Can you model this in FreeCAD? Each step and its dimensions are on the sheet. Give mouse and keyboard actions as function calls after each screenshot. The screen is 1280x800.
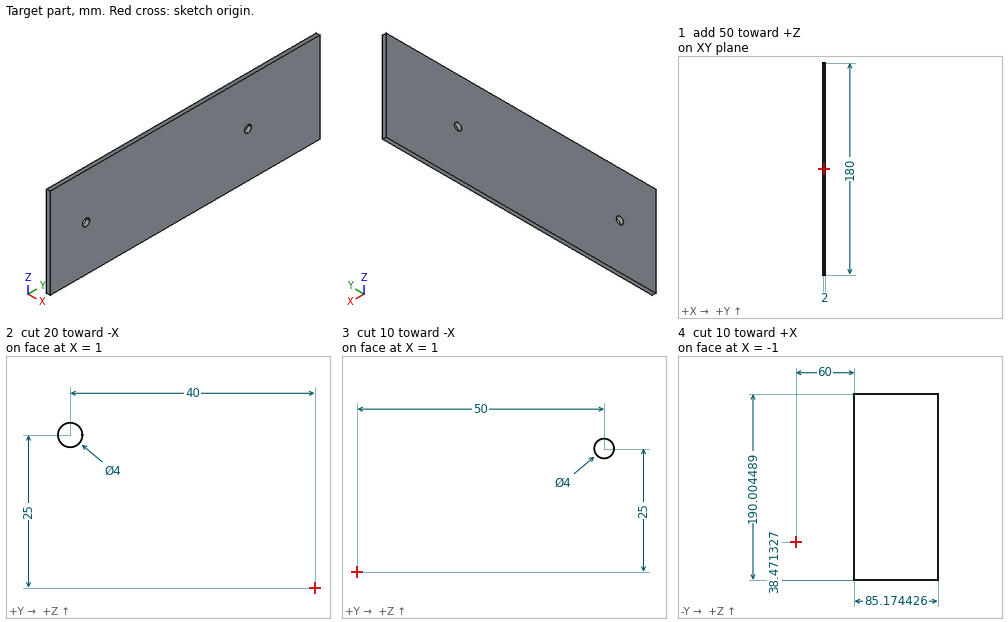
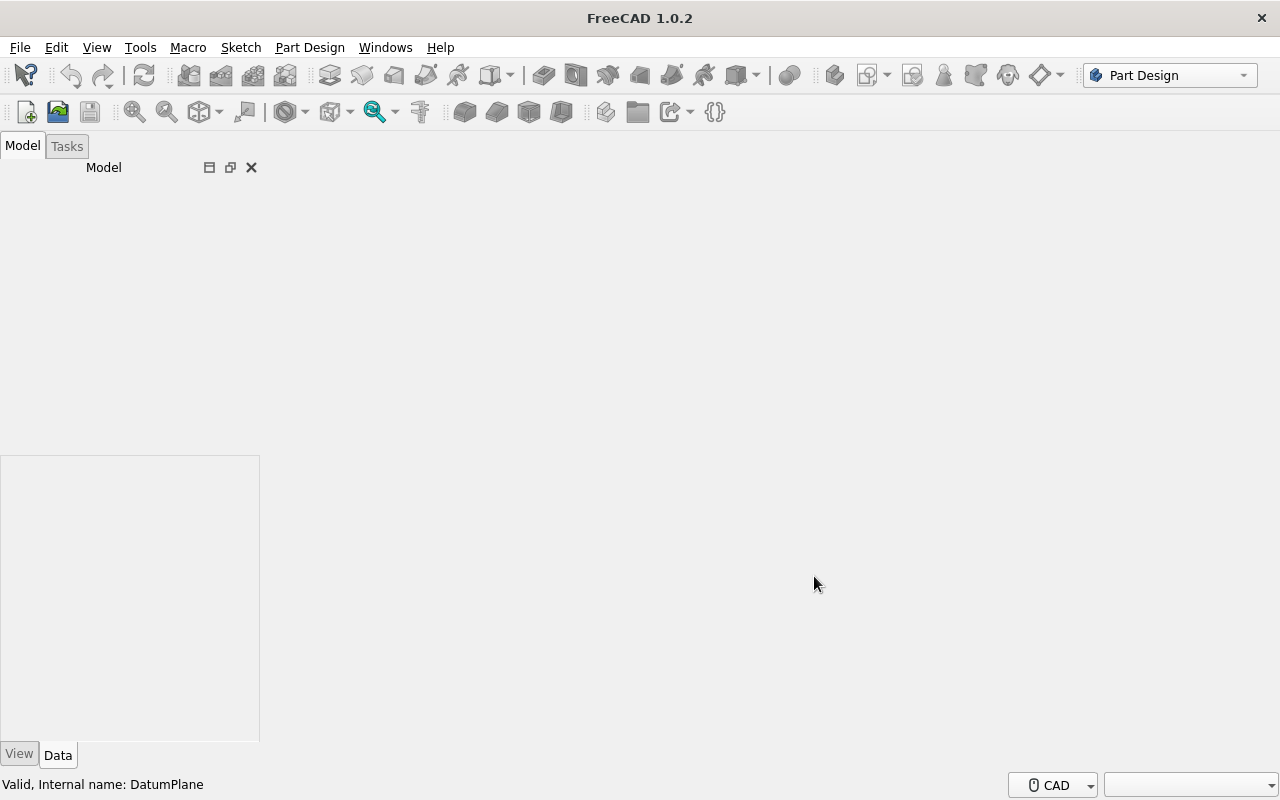
click(26, 112)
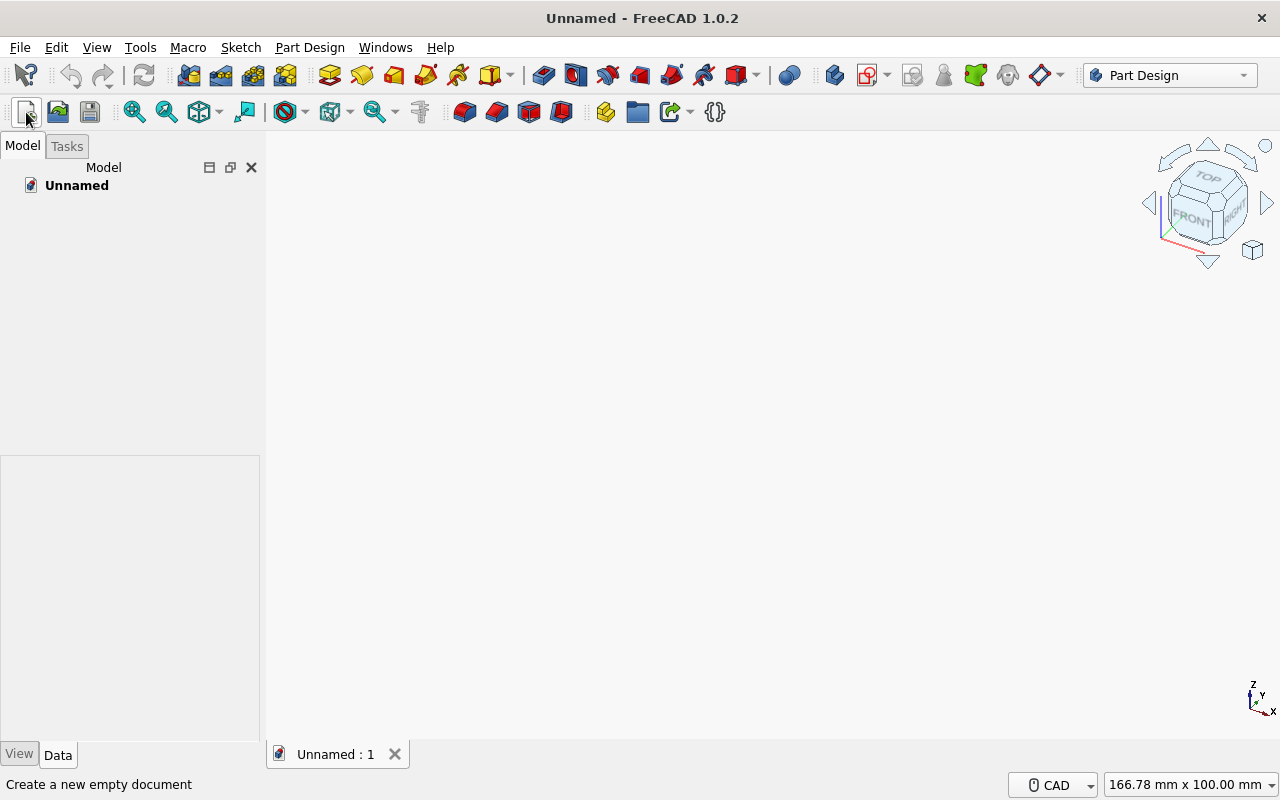
click(868, 76)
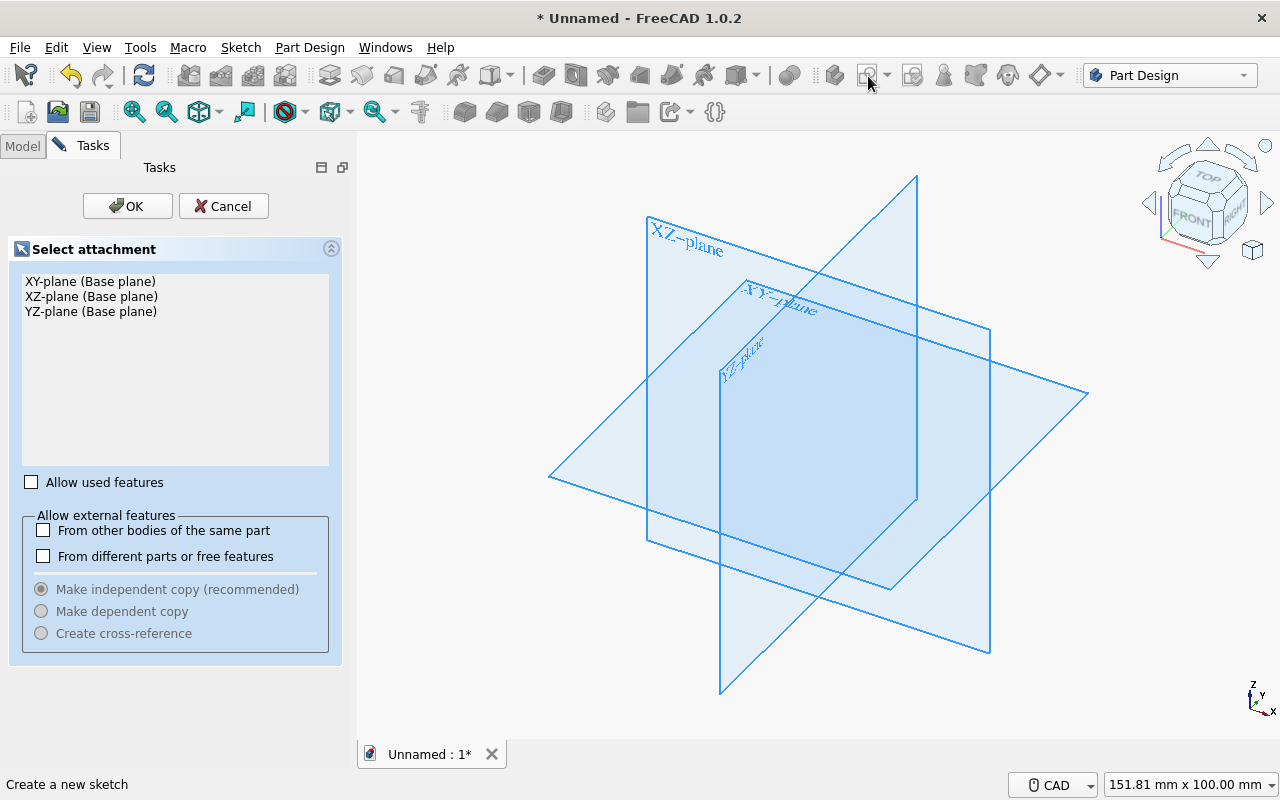
click(82, 282)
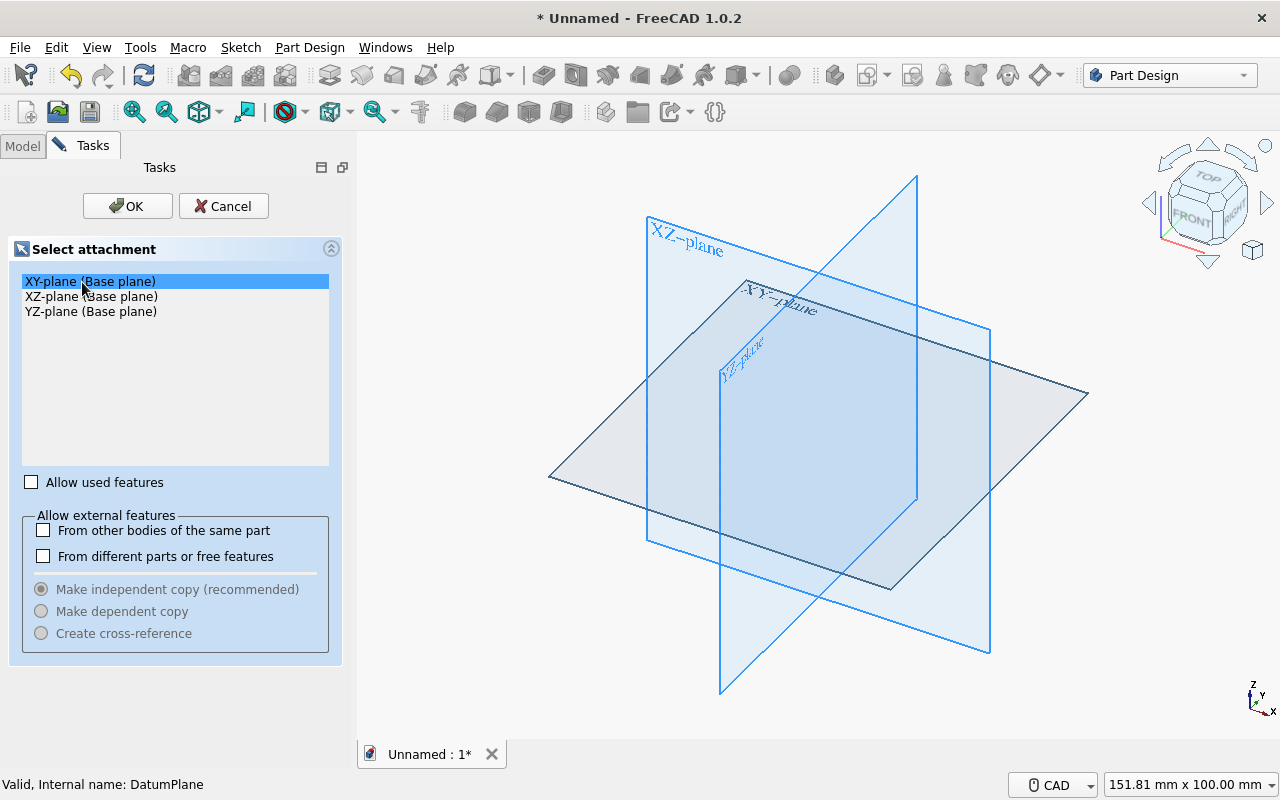
click(128, 206)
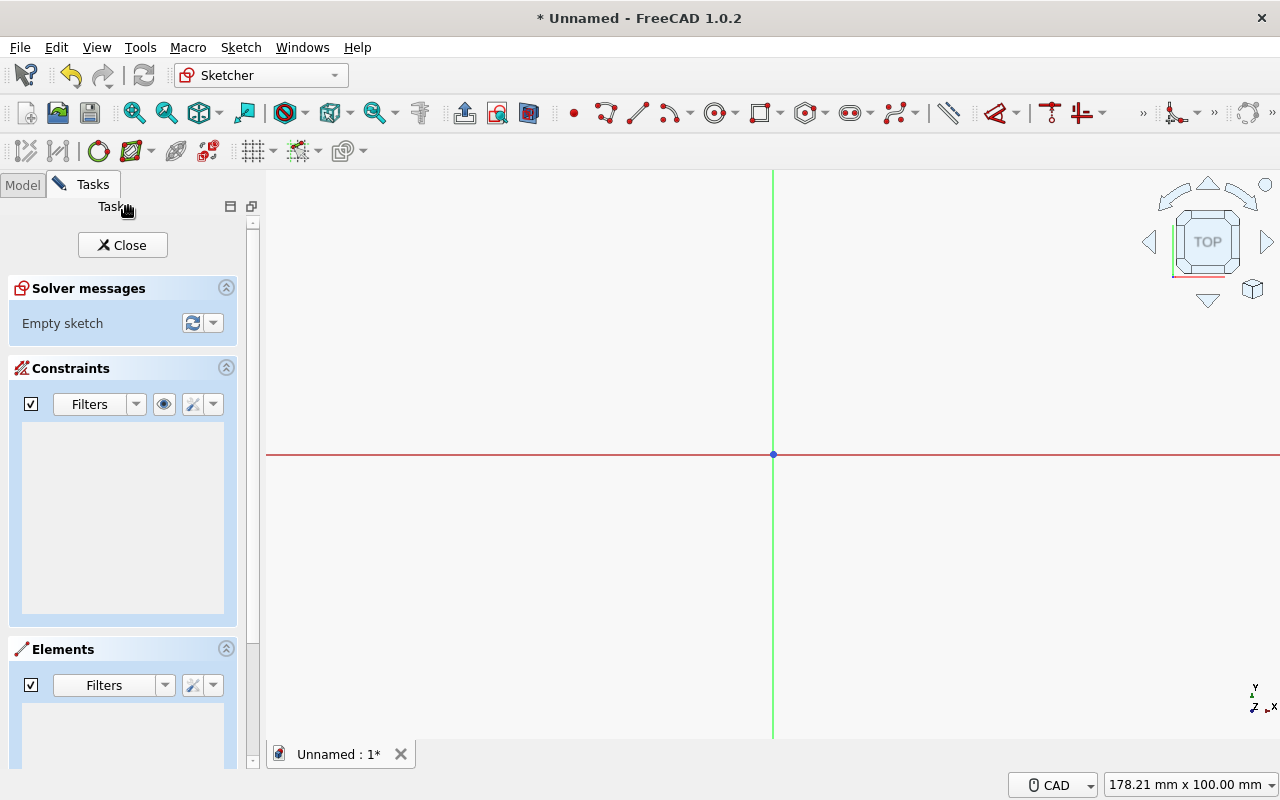
scroll(665, 454, down, 5)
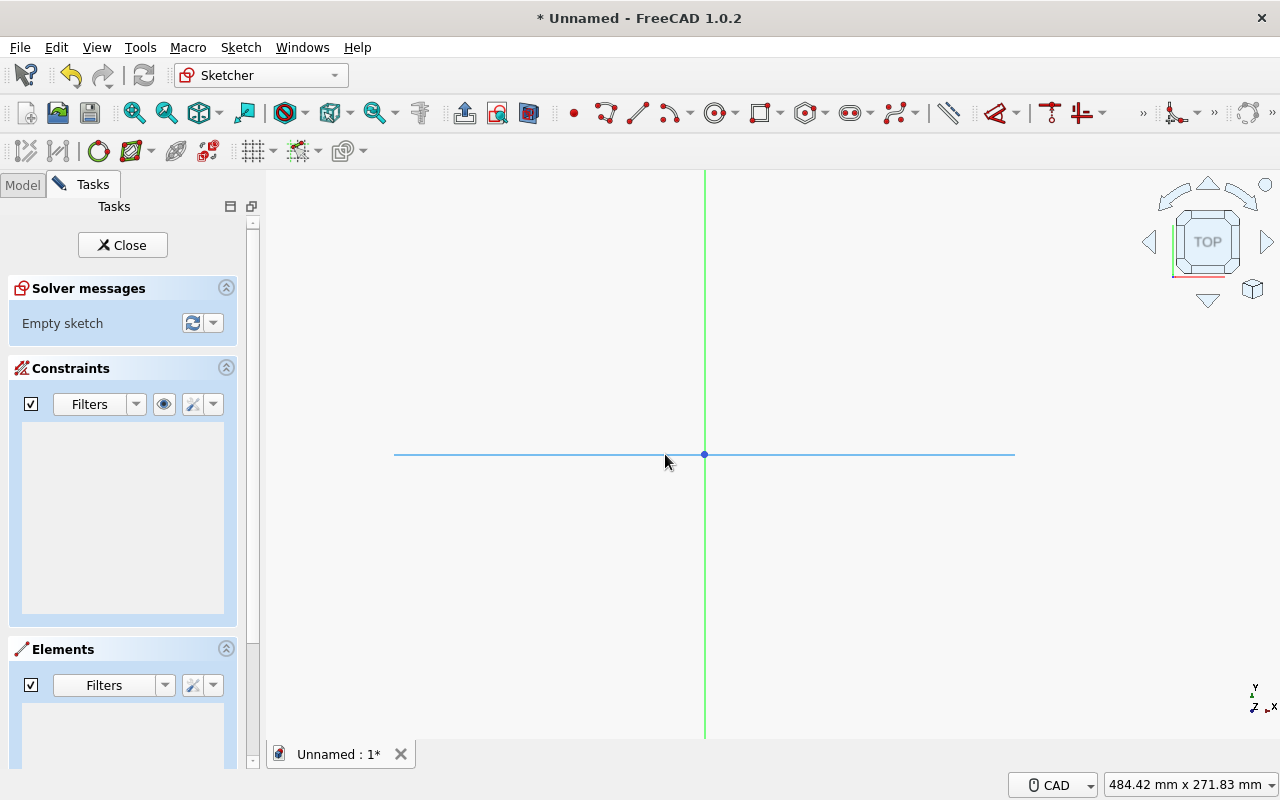
click(782, 114)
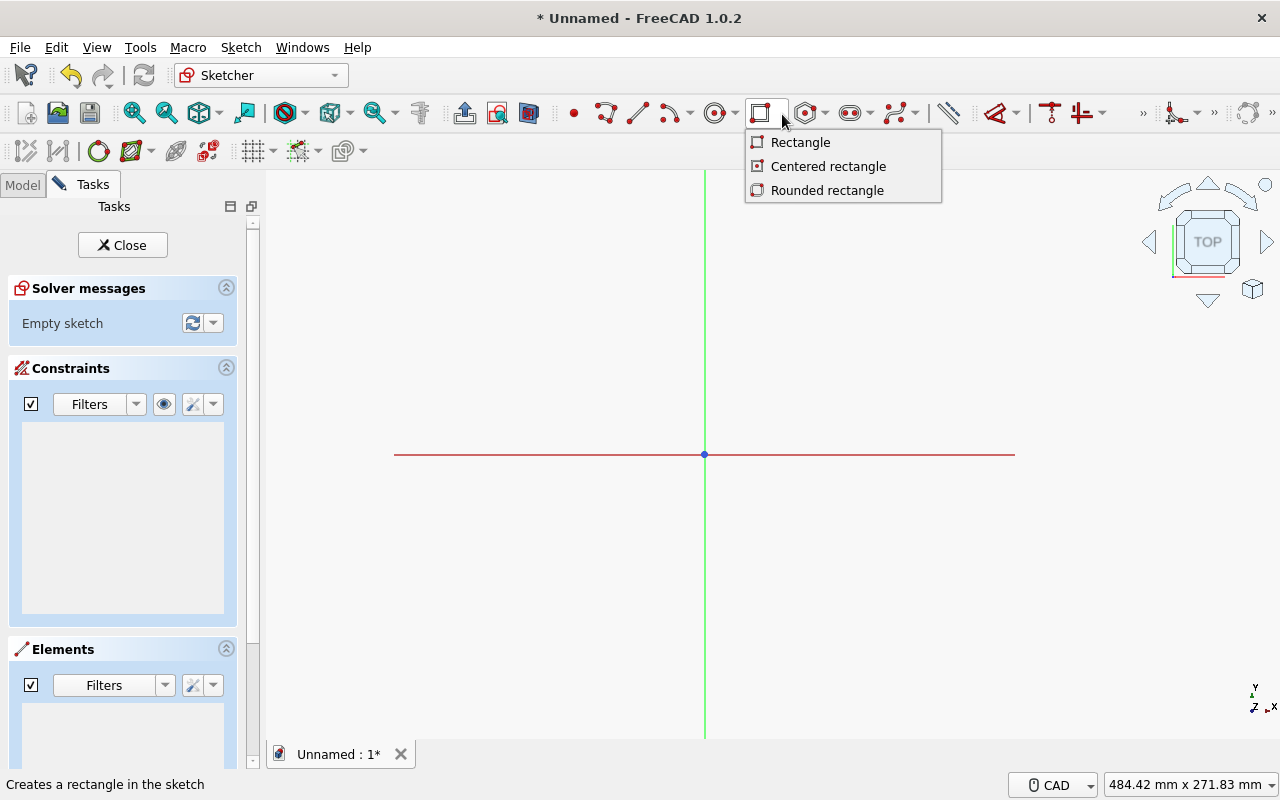
click(844, 166)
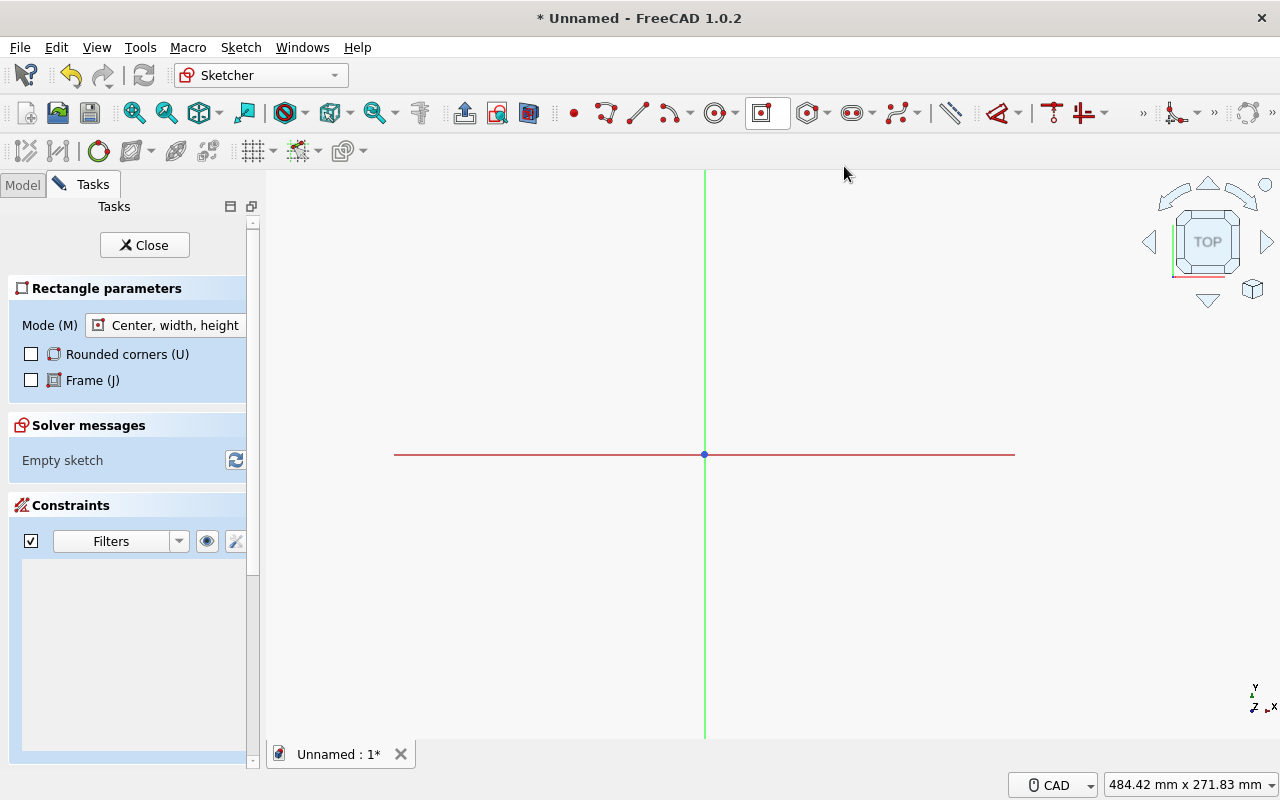
scroll(705, 454, up, 11)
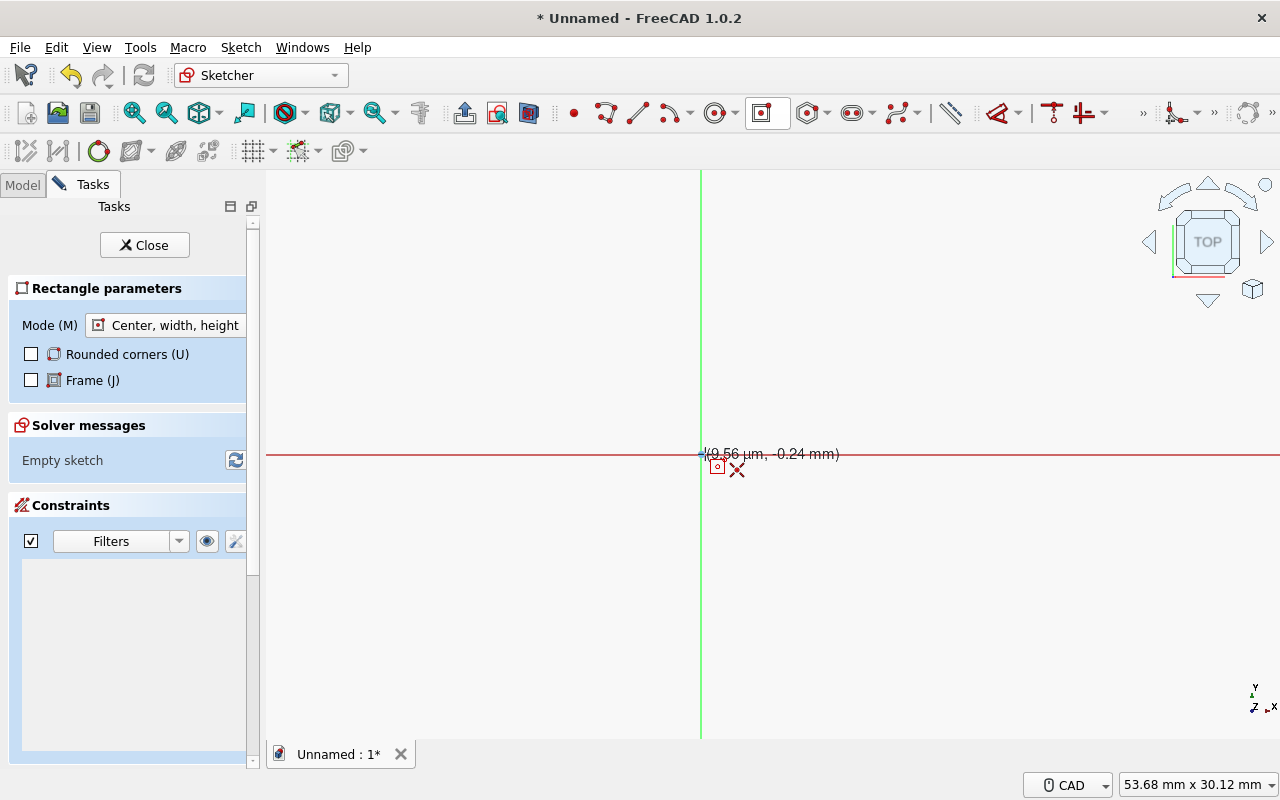
scroll(705, 454, down, 11)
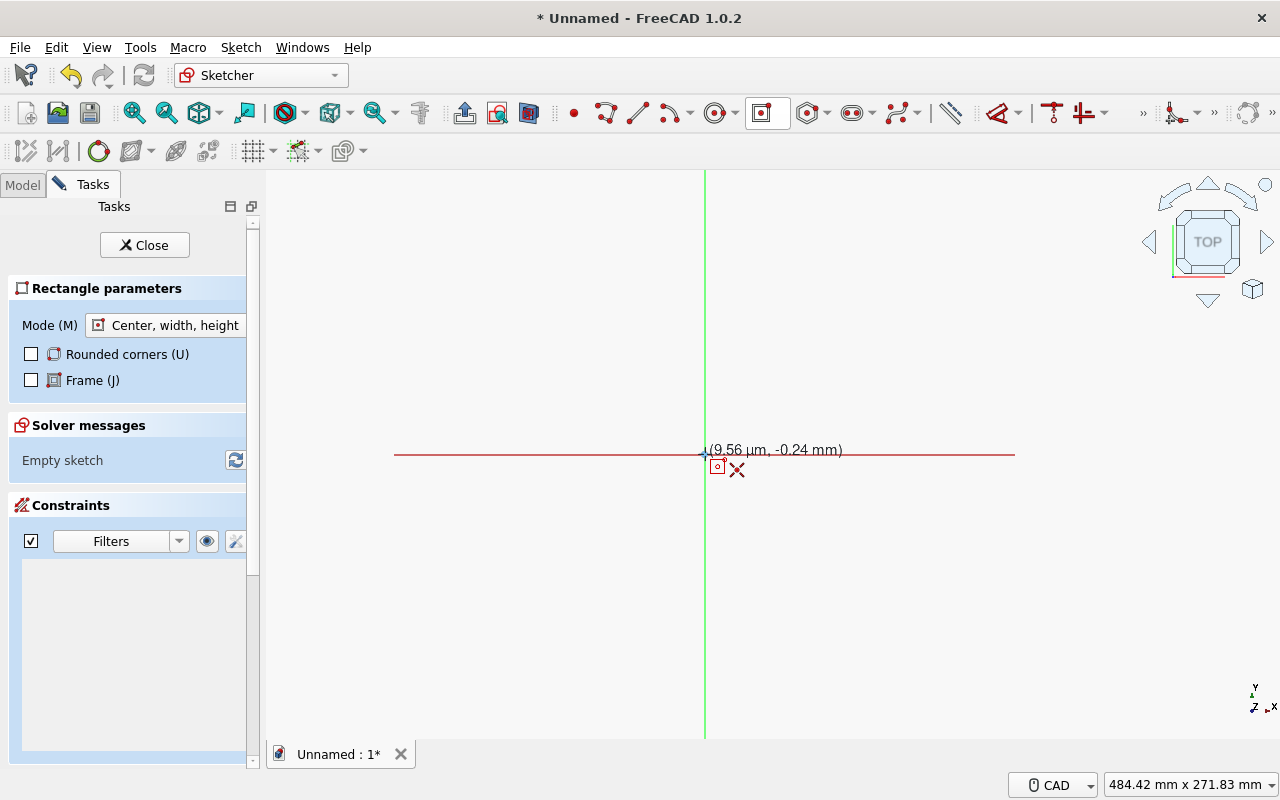
click(705, 454)